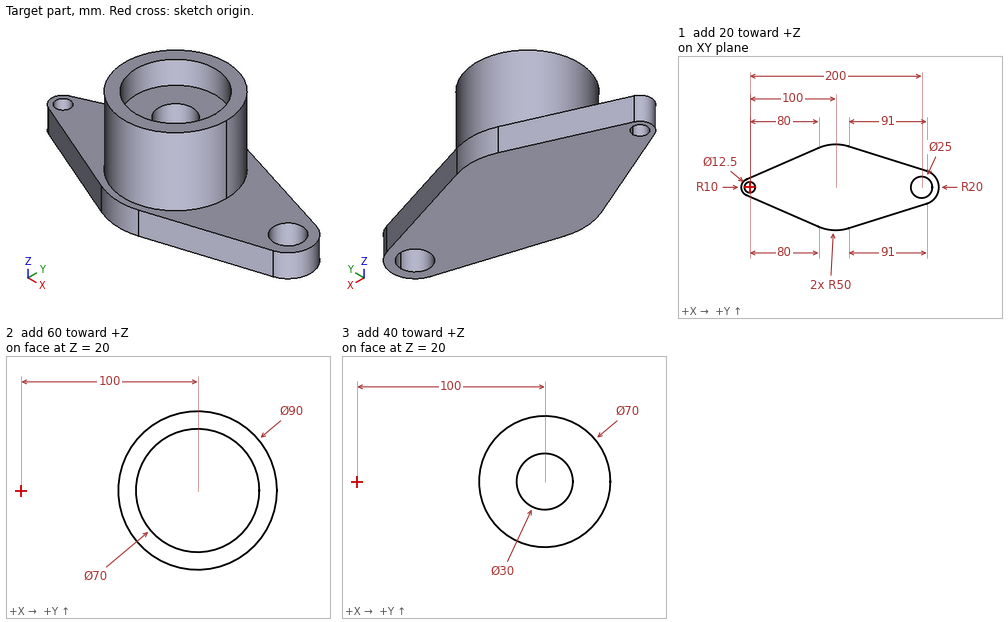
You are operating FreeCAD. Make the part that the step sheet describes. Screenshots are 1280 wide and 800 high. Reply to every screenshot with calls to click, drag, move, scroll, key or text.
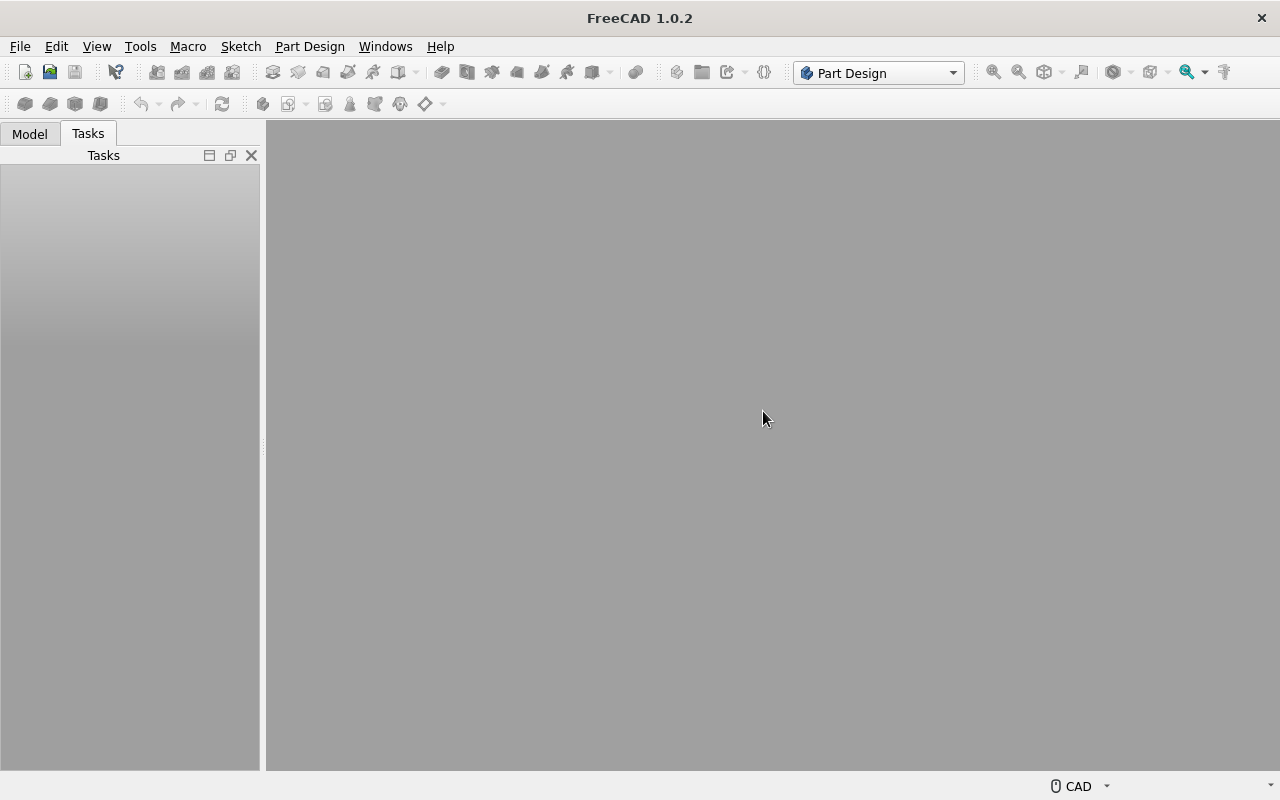
click(25, 72)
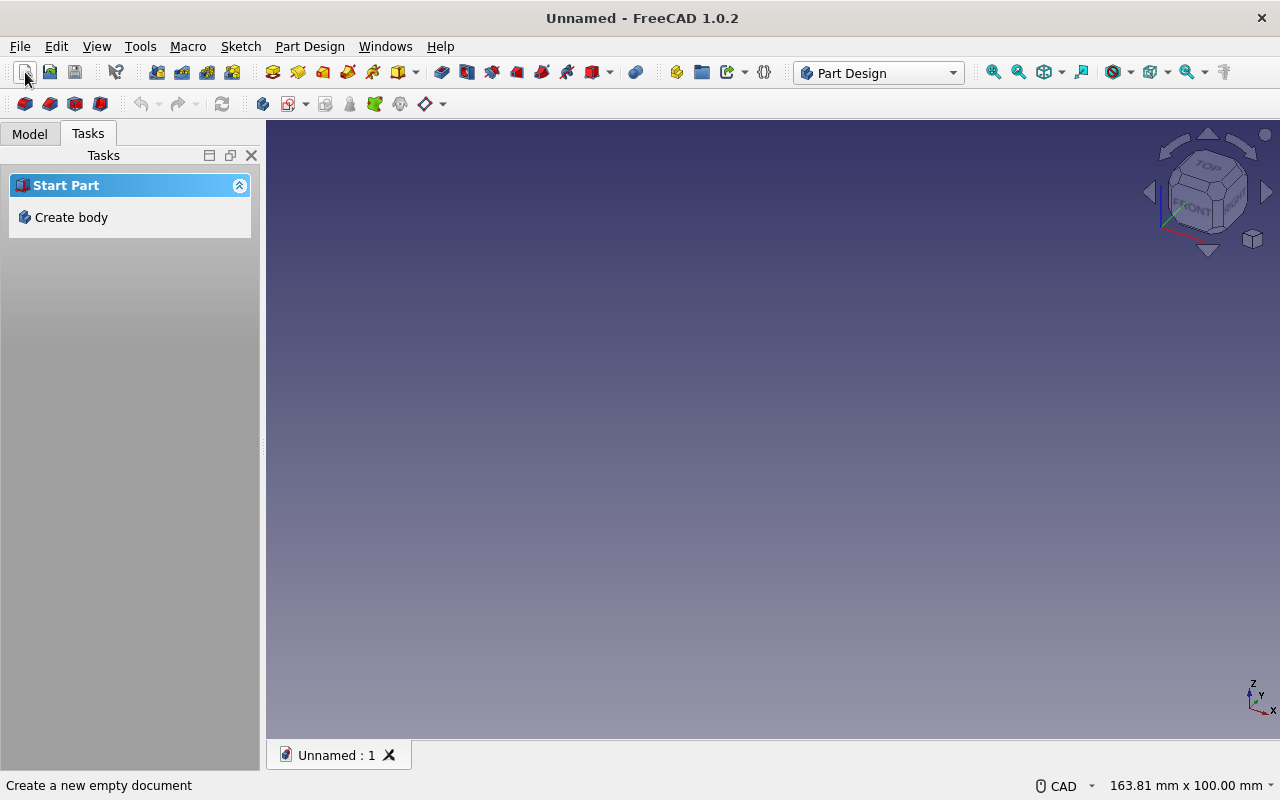
click(288, 104)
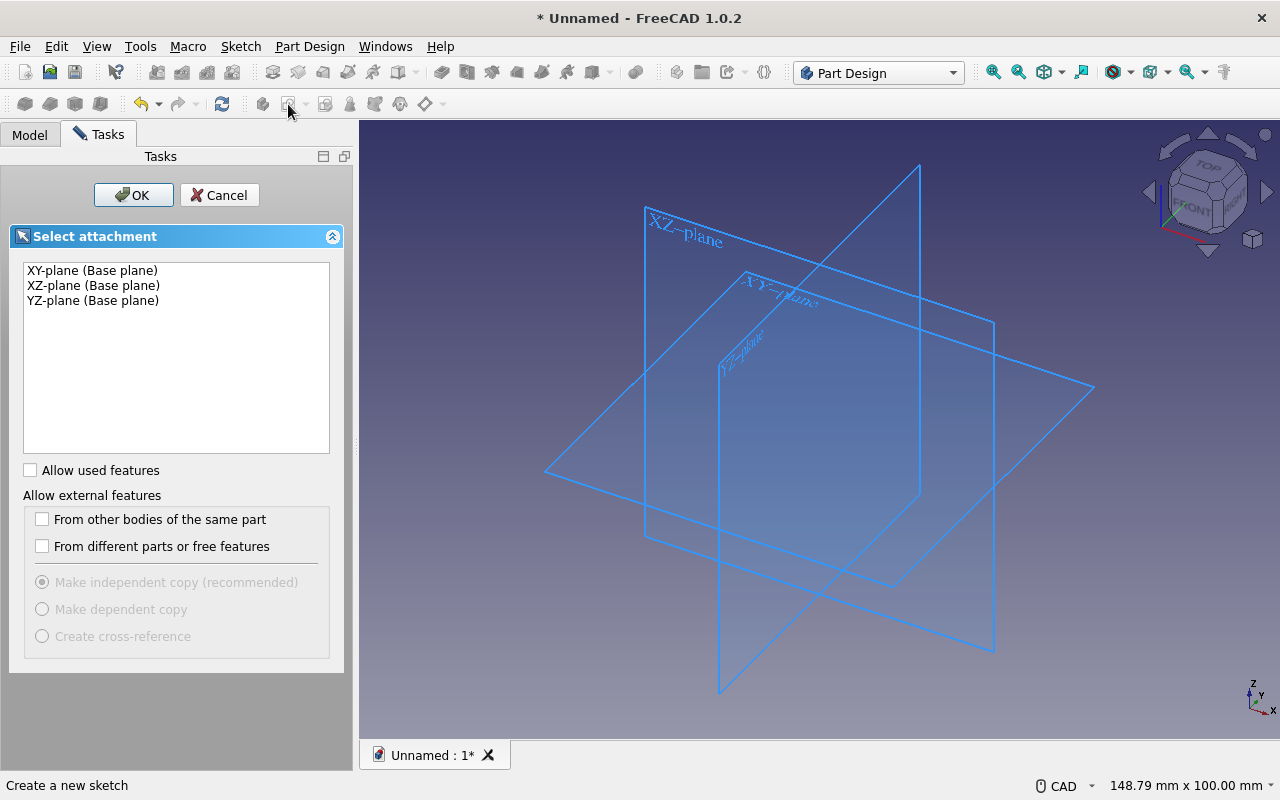
click(84, 270)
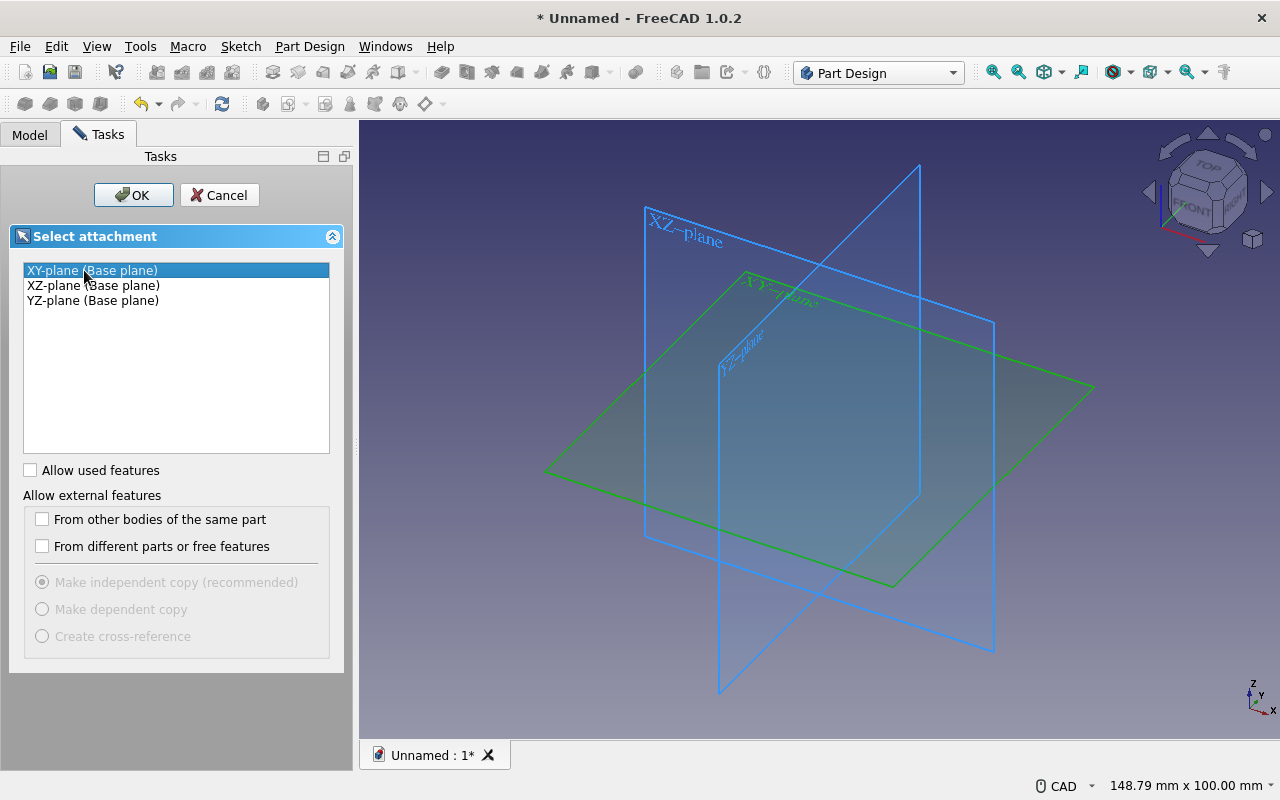
click(134, 195)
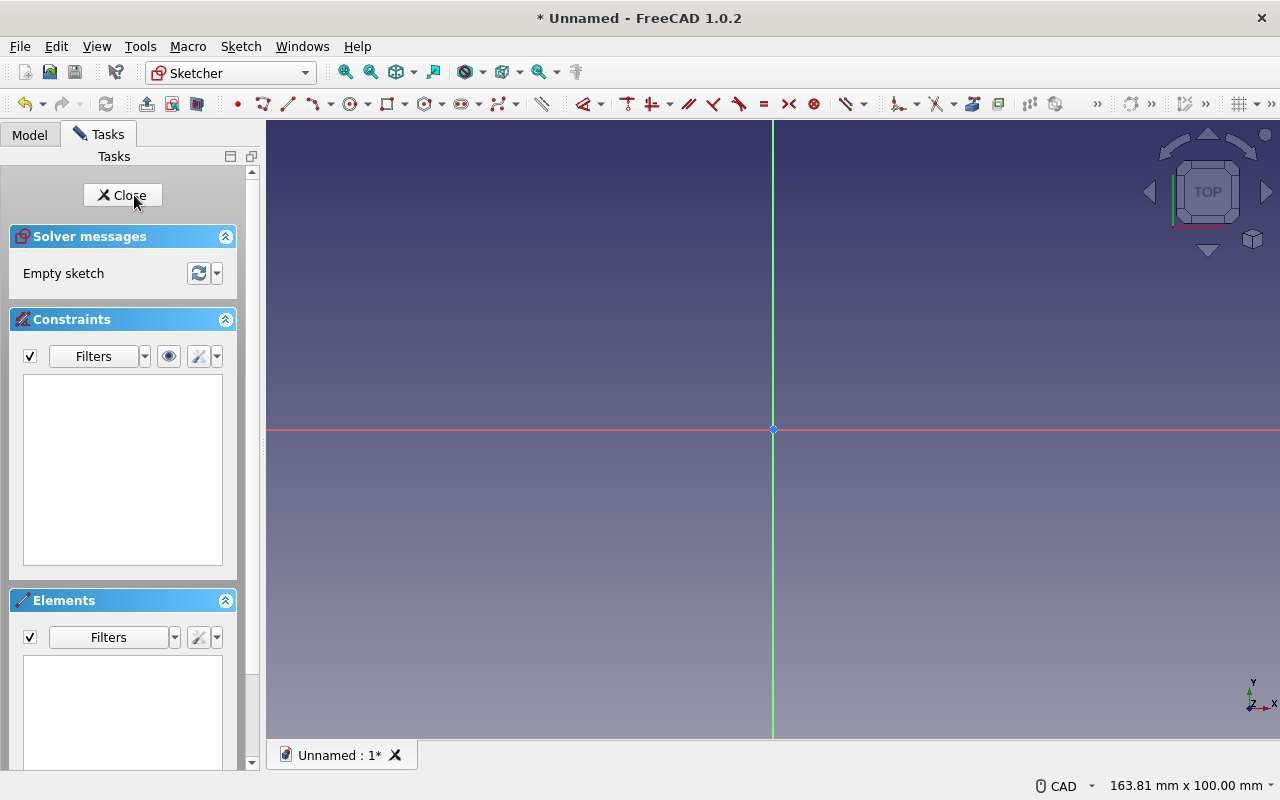
scroll(294, 430, down, 5)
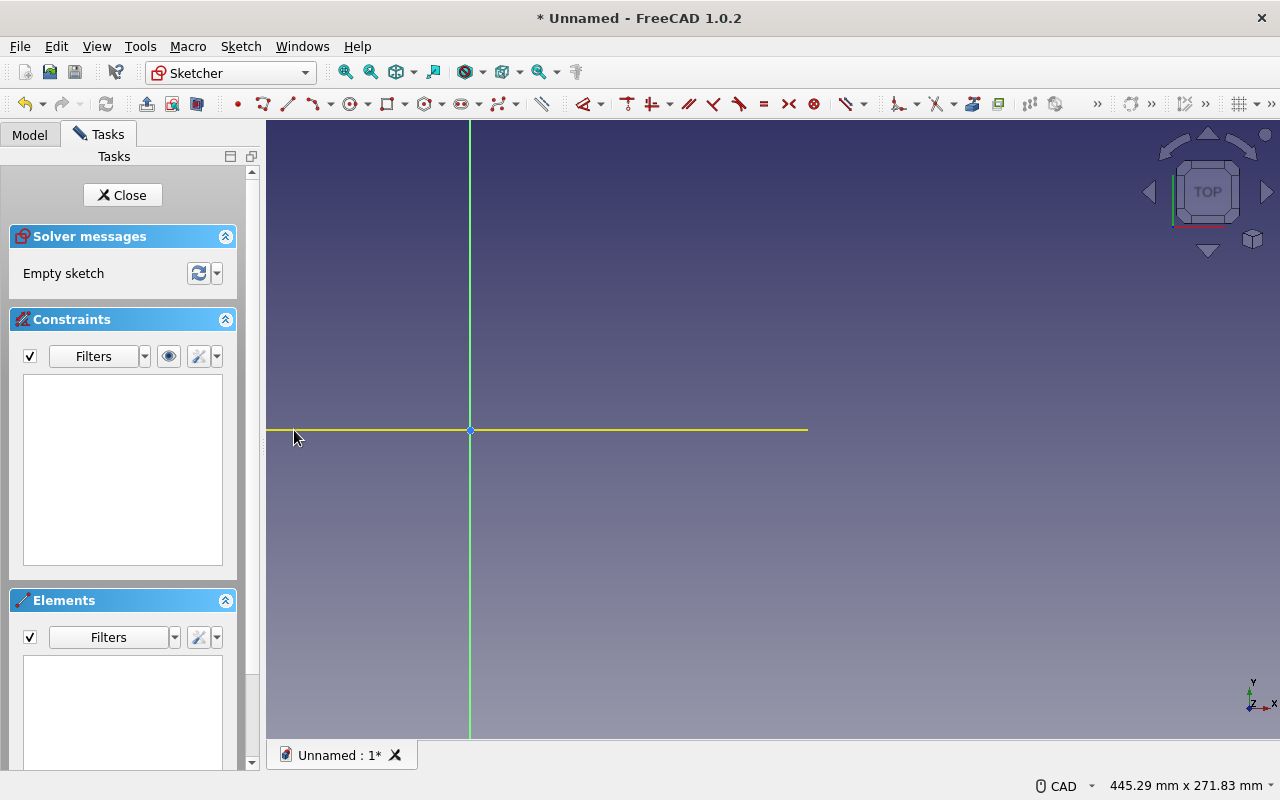
click(288, 104)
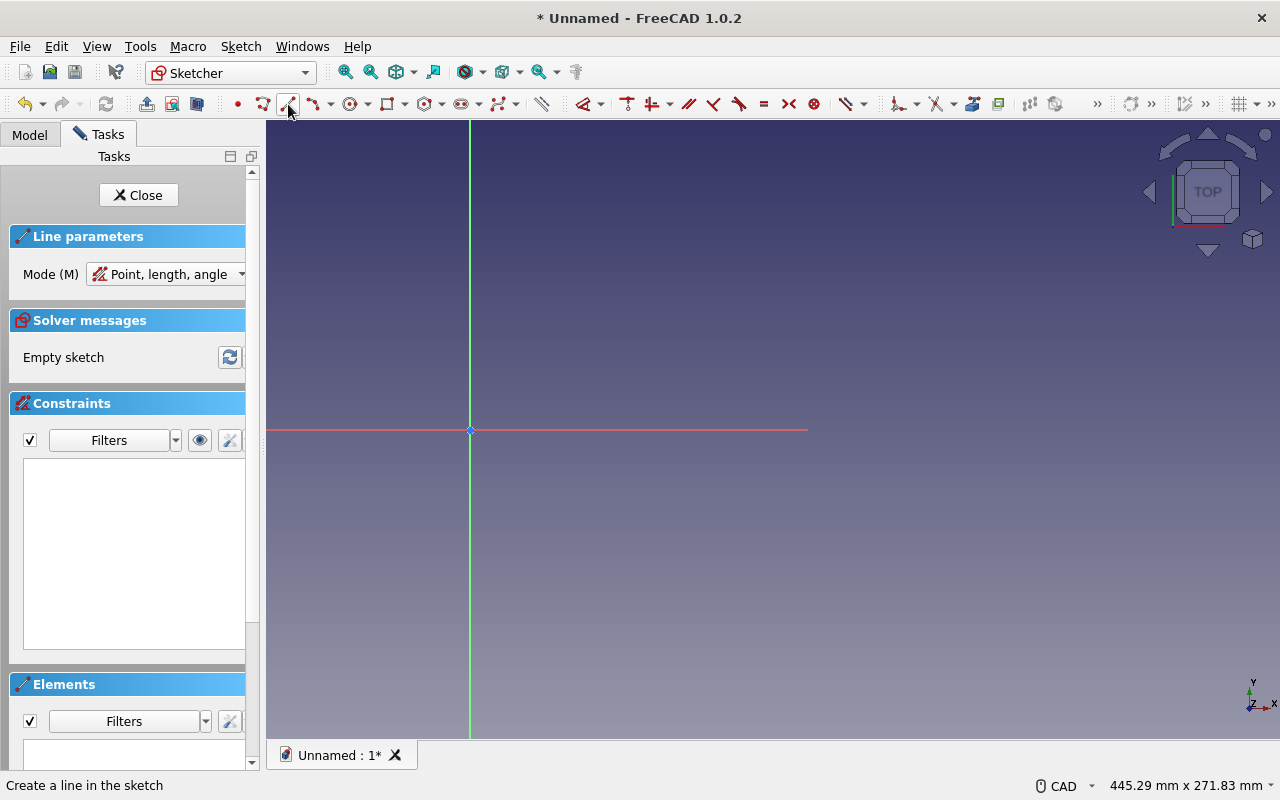
click(652, 326)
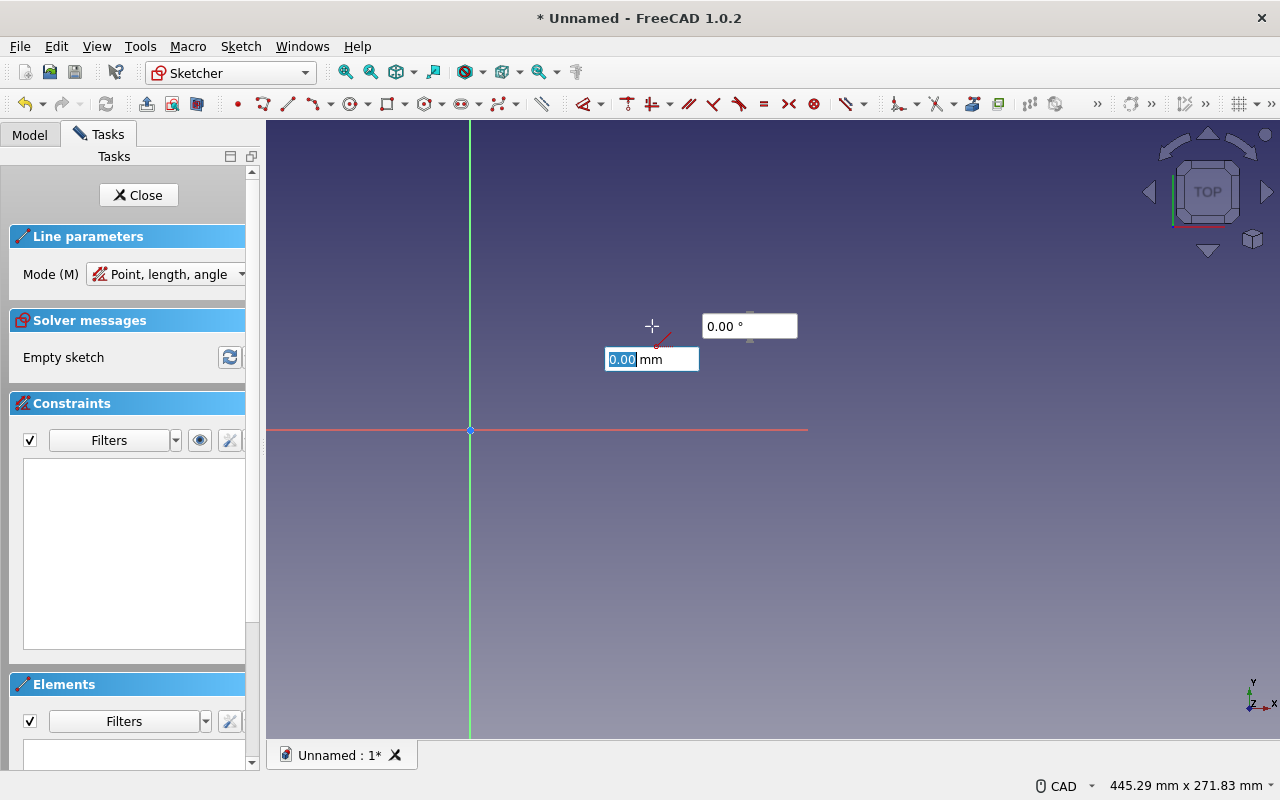
scroll(461, 409, up, 3)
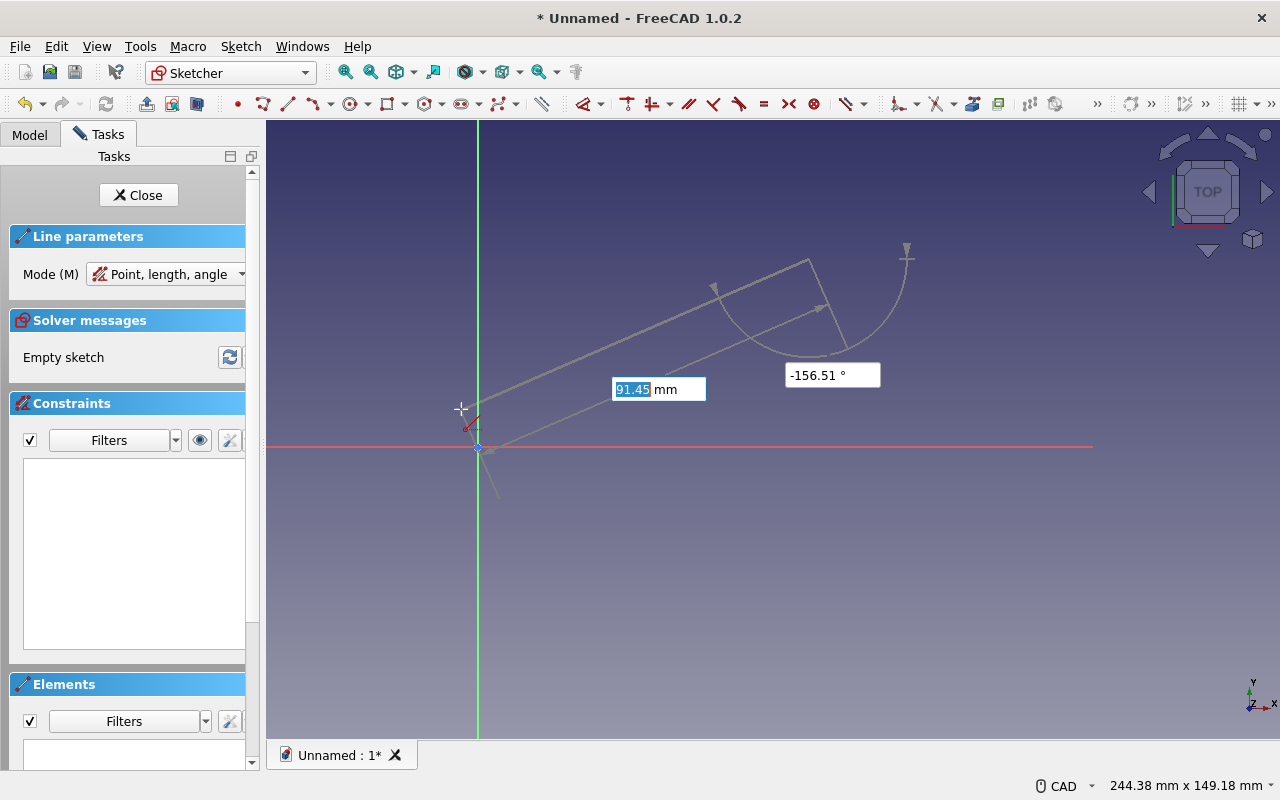
click(461, 409)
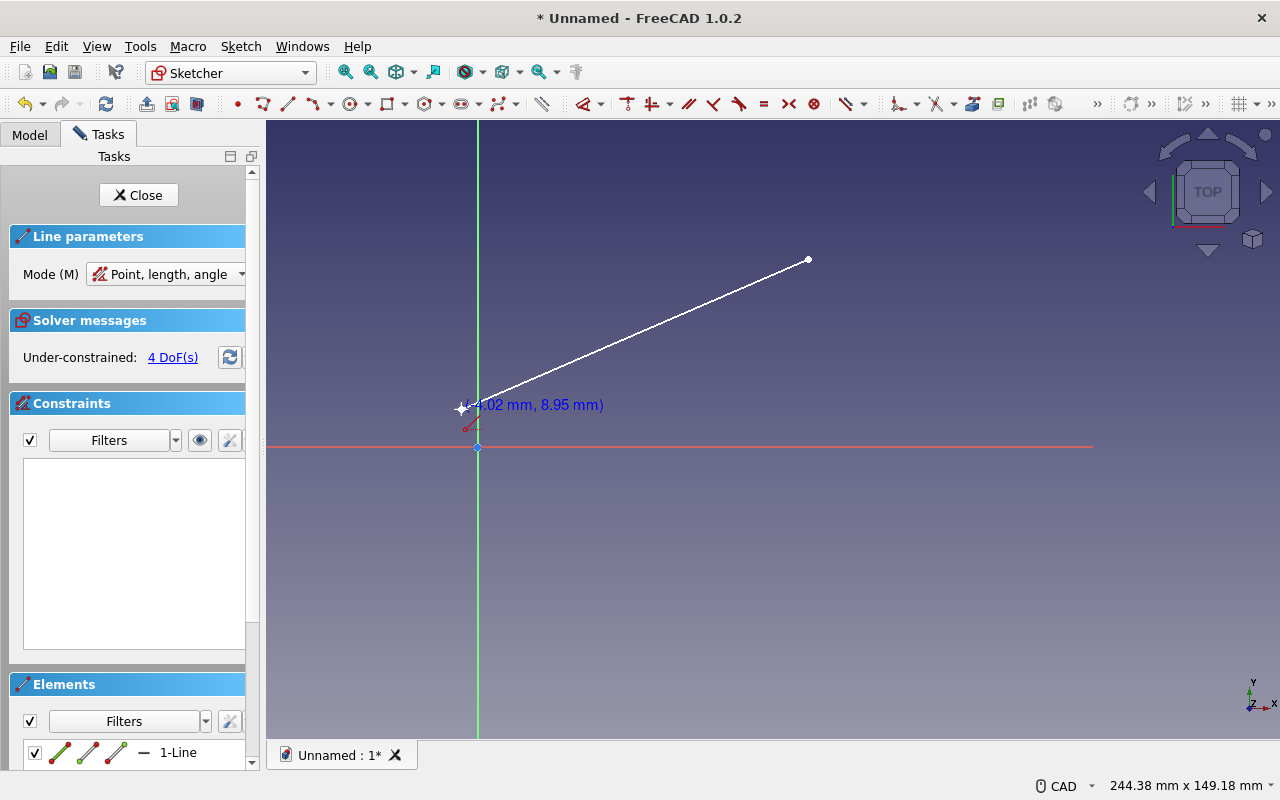
click(461, 485)
click(810, 637)